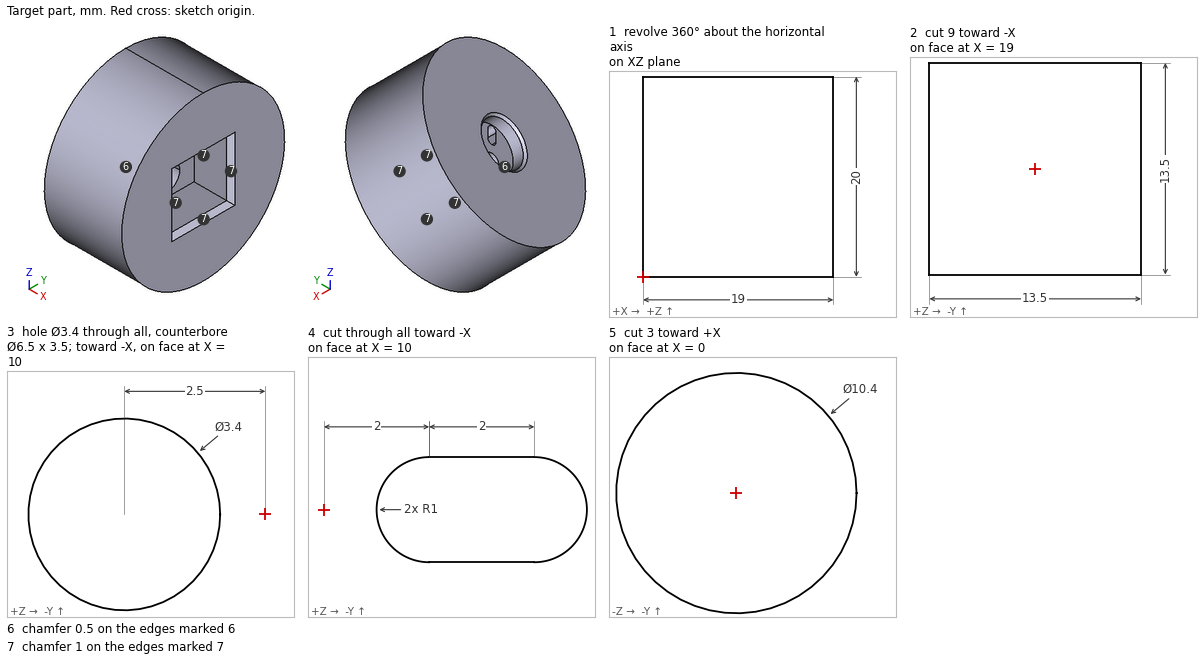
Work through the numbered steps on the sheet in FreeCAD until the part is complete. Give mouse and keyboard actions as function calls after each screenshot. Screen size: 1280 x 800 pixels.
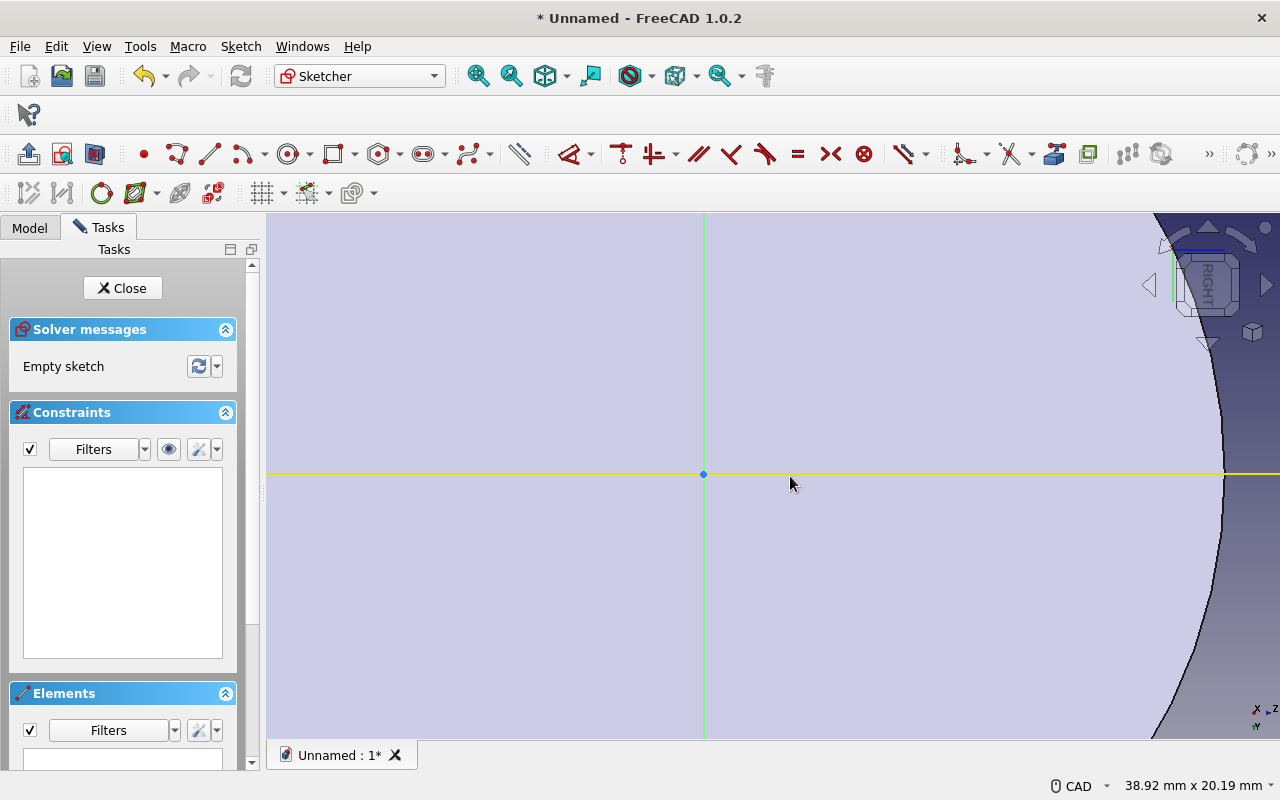
click(354, 154)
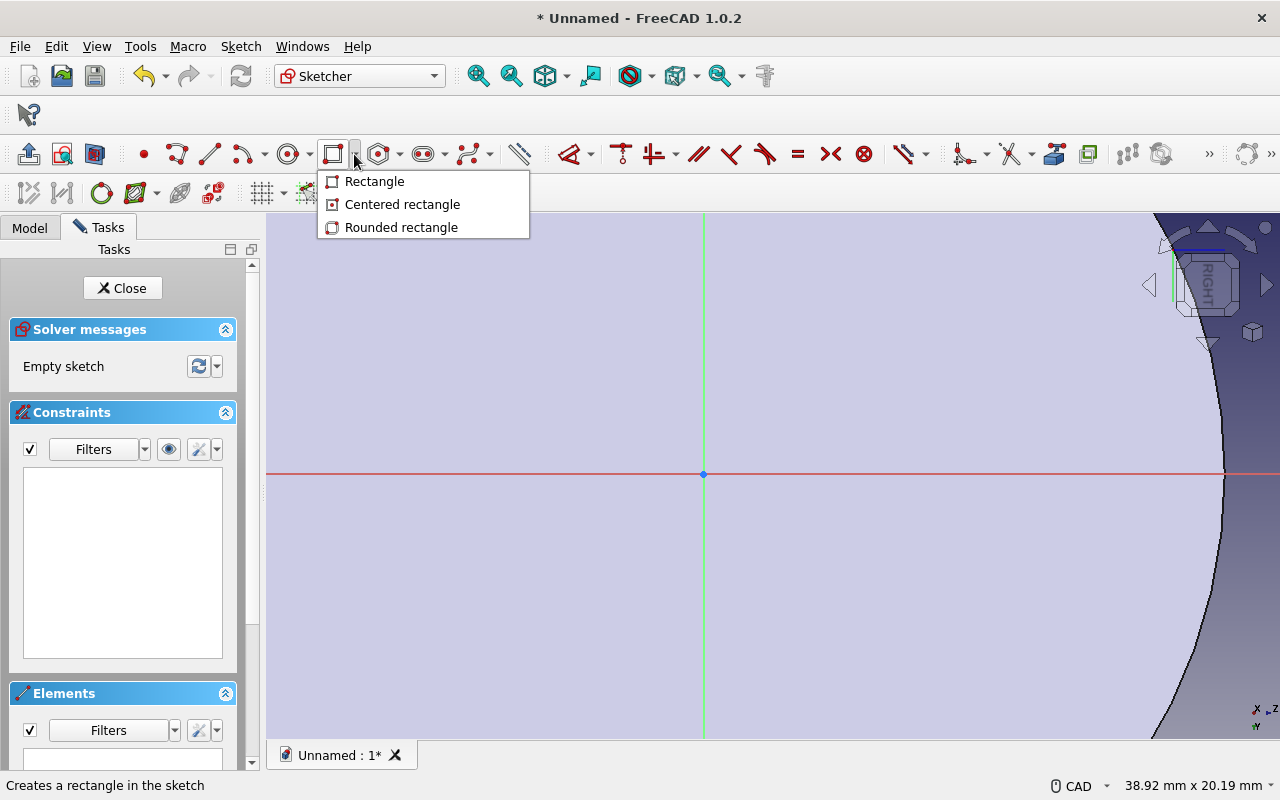
click(424, 204)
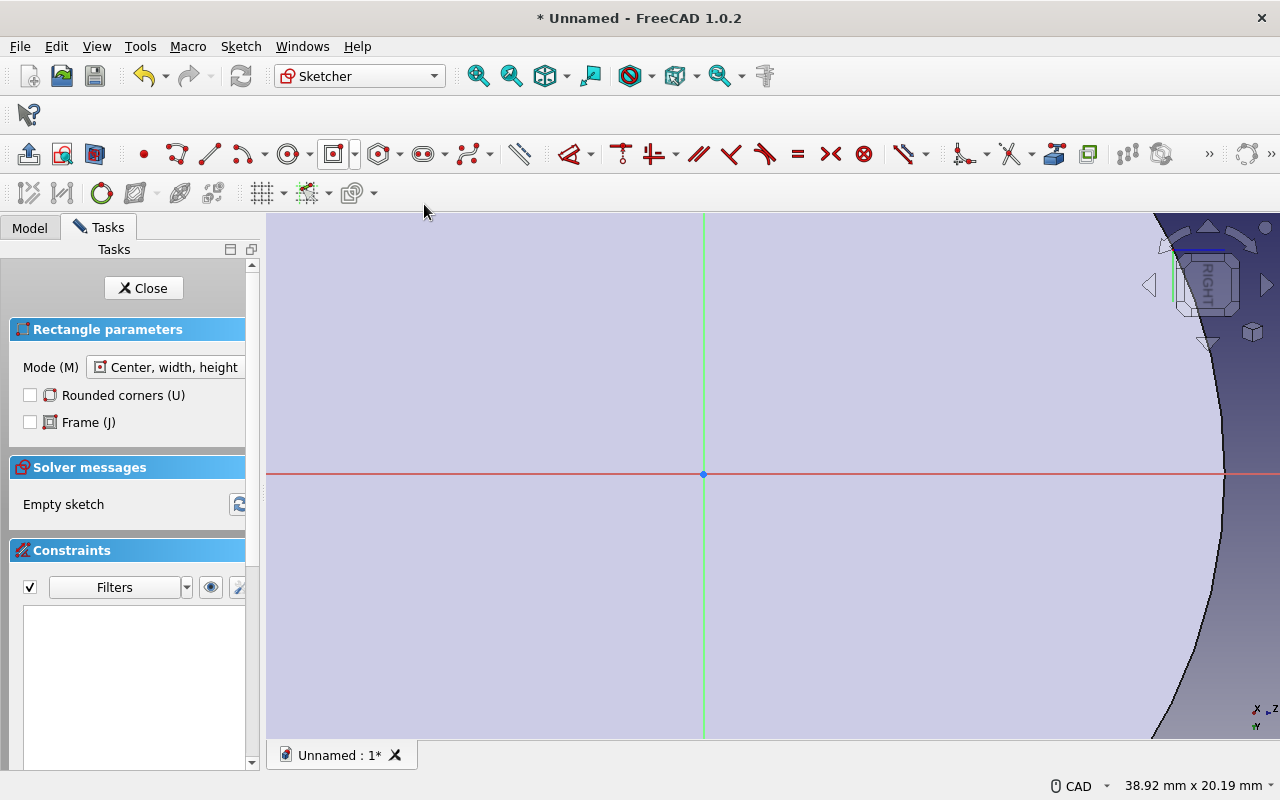
click(704, 474)
click(880, 298)
key(Escape)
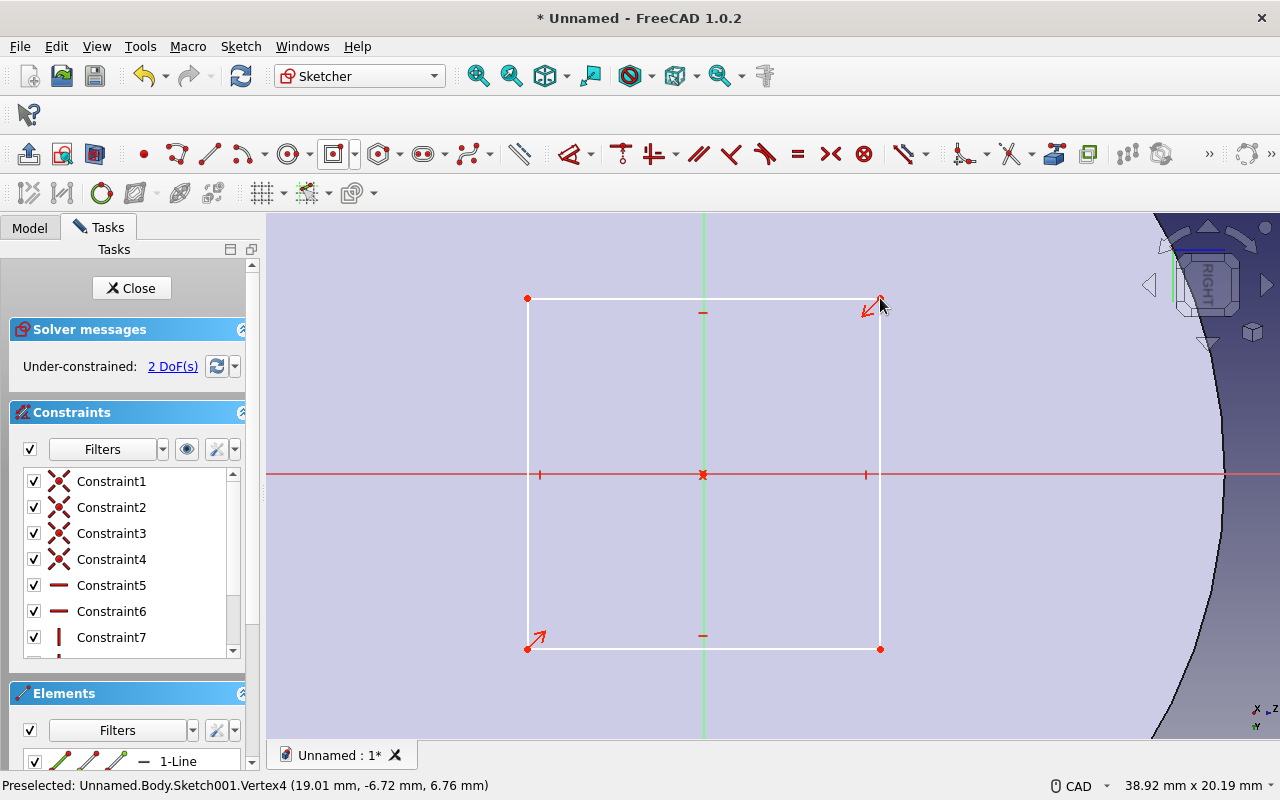
click(568, 154)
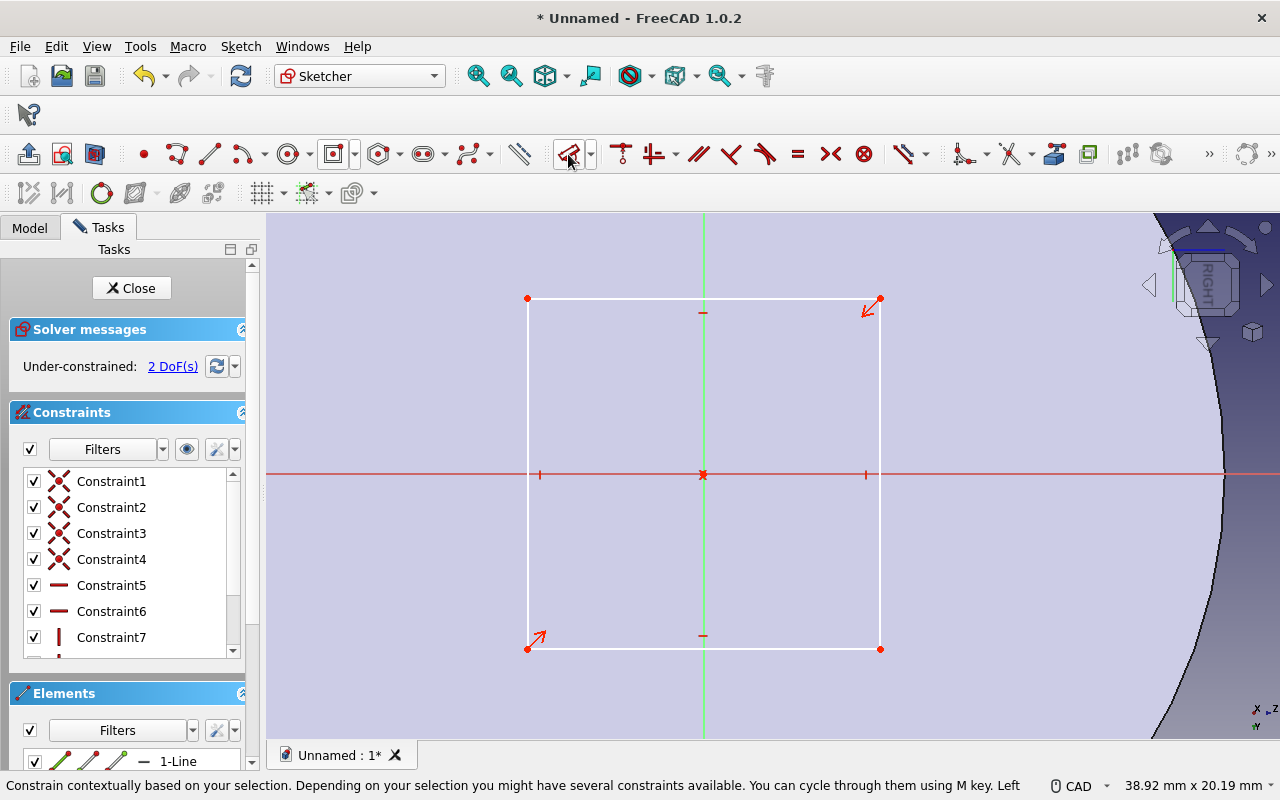
click(633, 649)
click(623, 683)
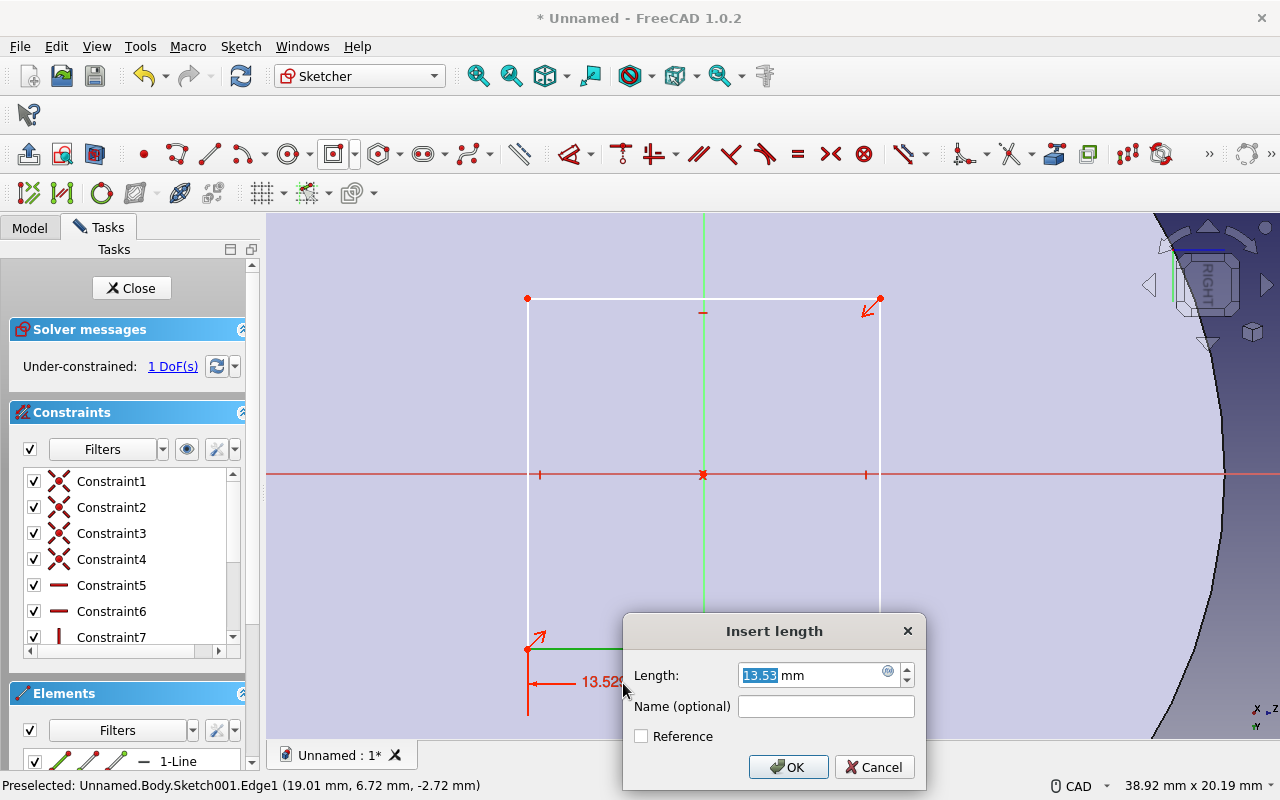
text(13.5)
key(Return)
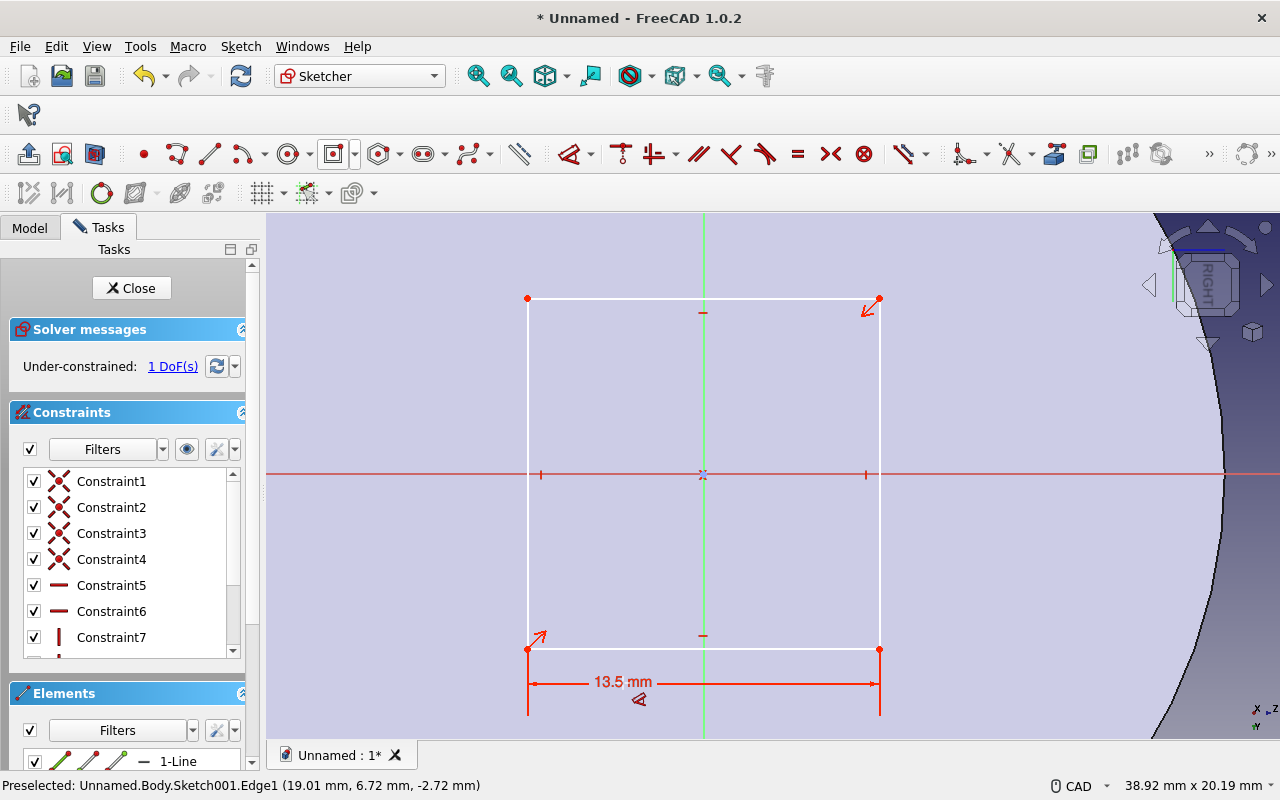
click(880, 544)
click(914, 394)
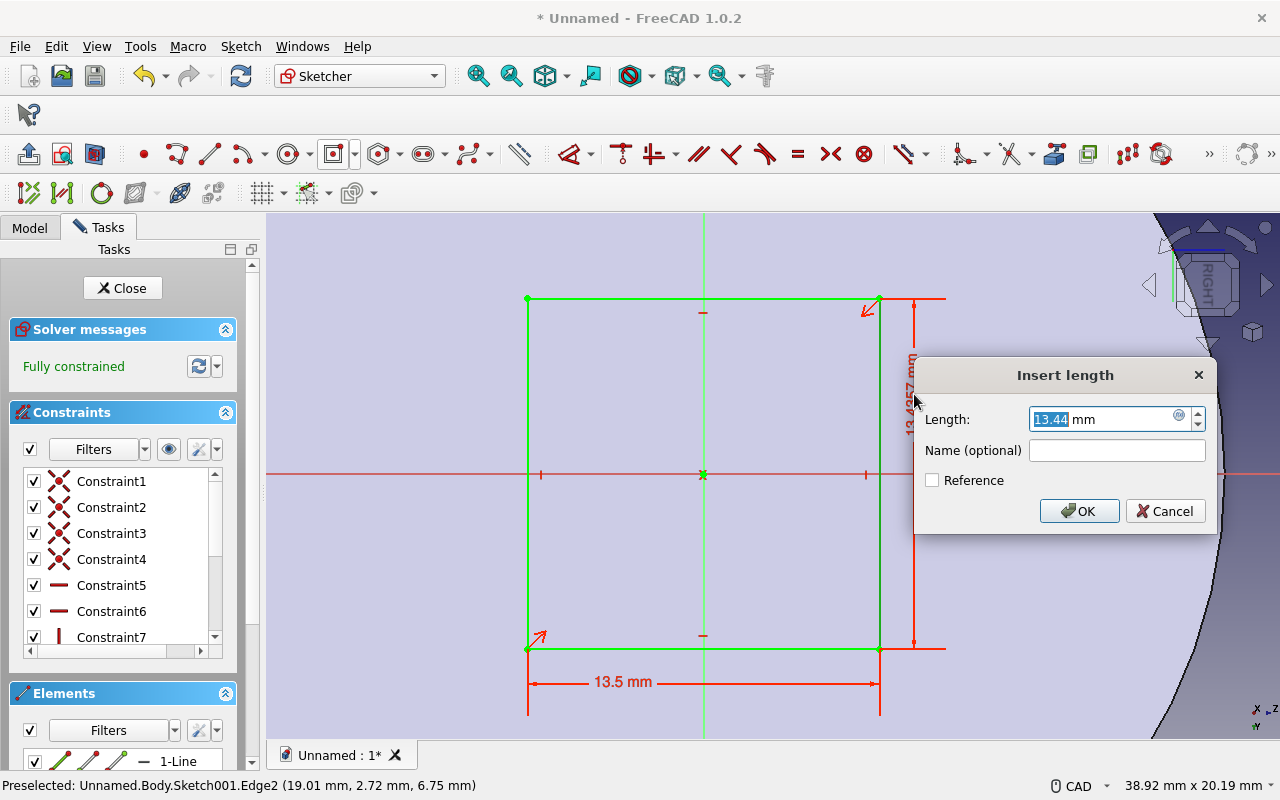
text(13.5)
key(Return)
key(Escape)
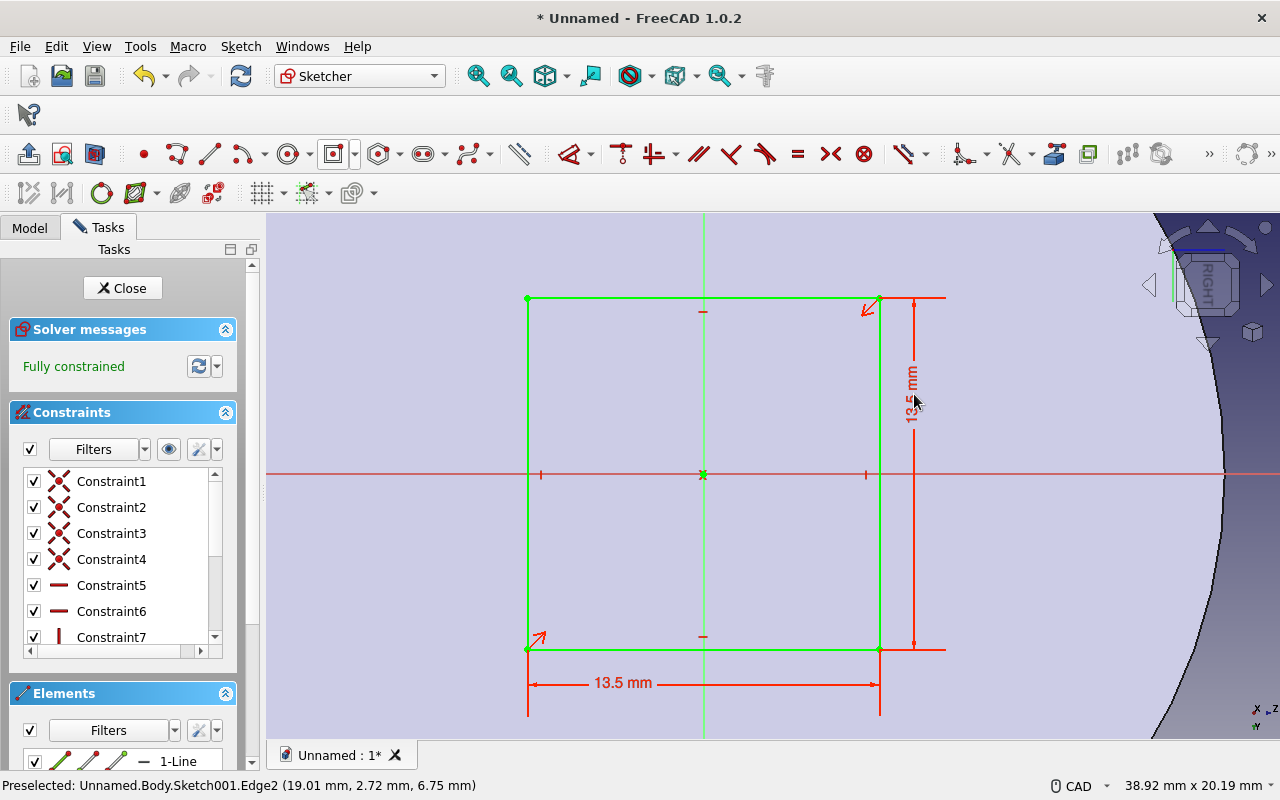
click(123, 288)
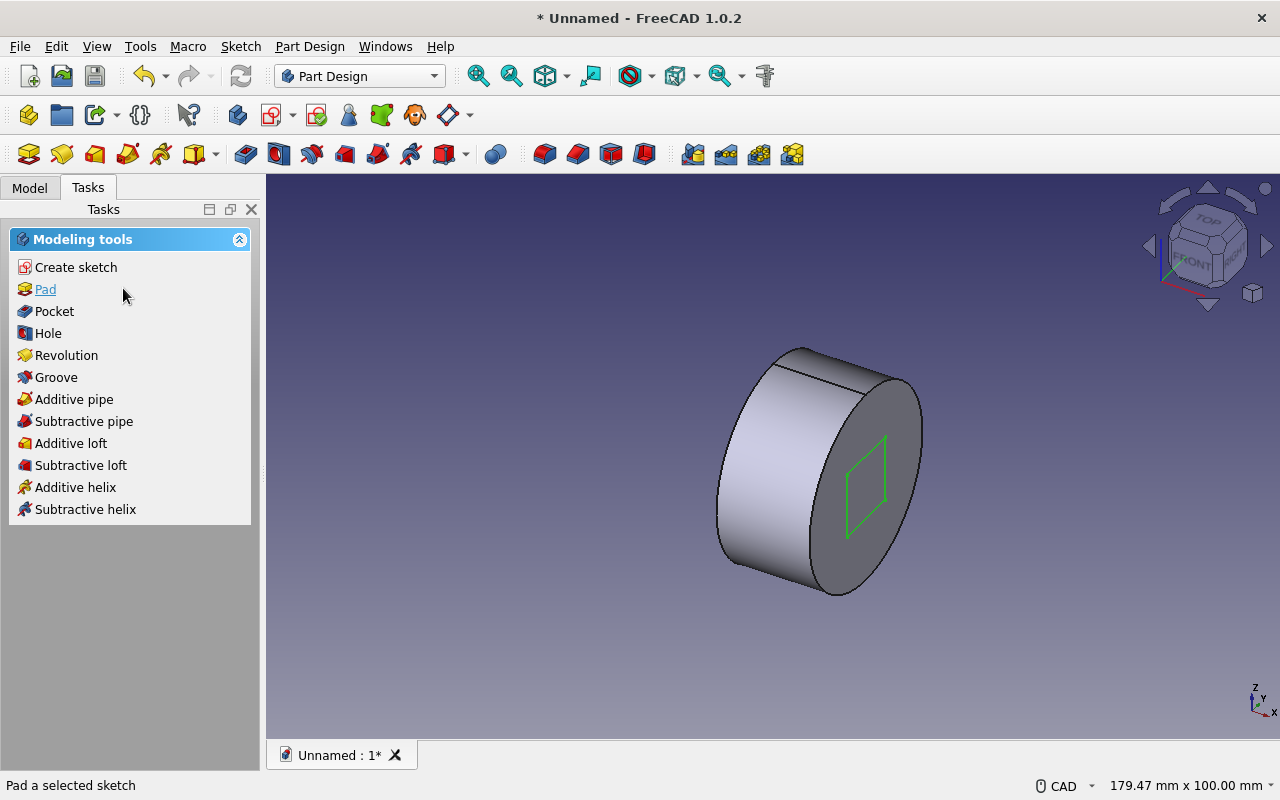
click(246, 154)